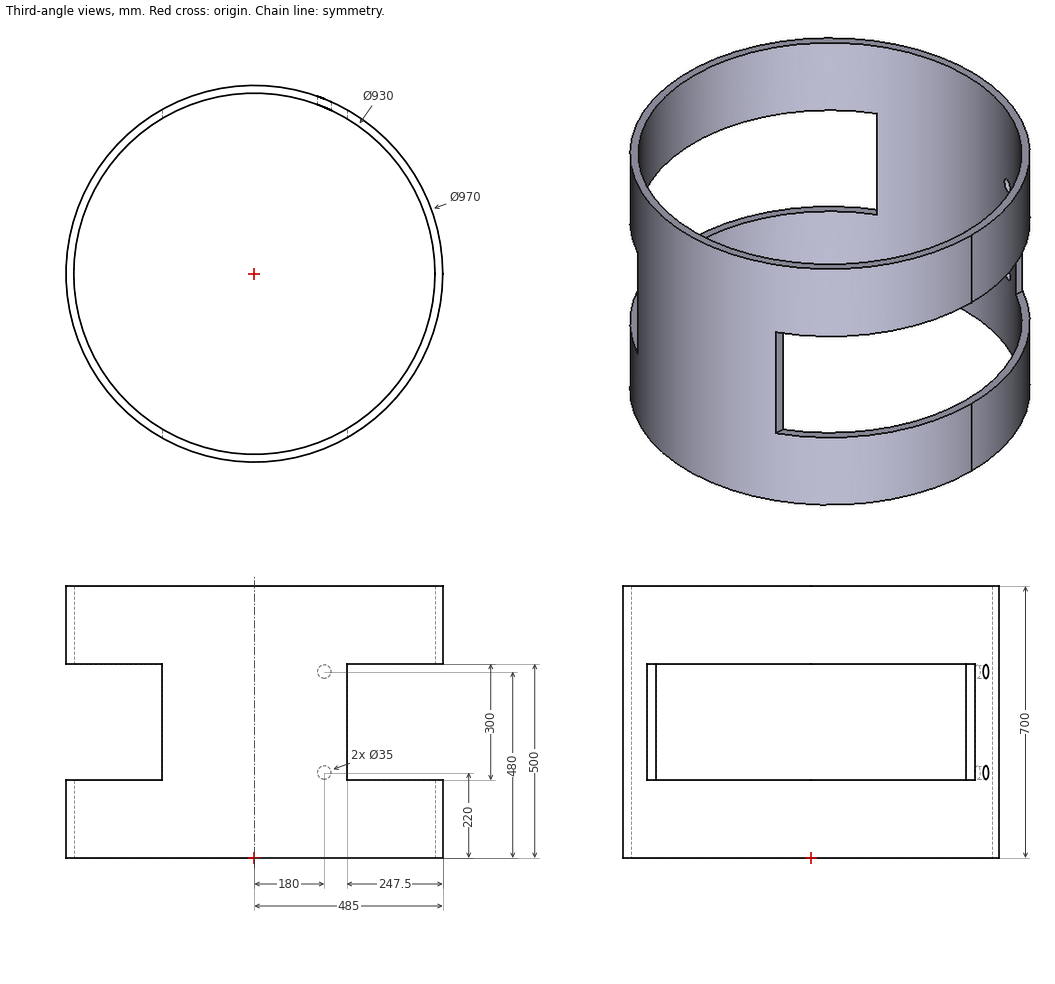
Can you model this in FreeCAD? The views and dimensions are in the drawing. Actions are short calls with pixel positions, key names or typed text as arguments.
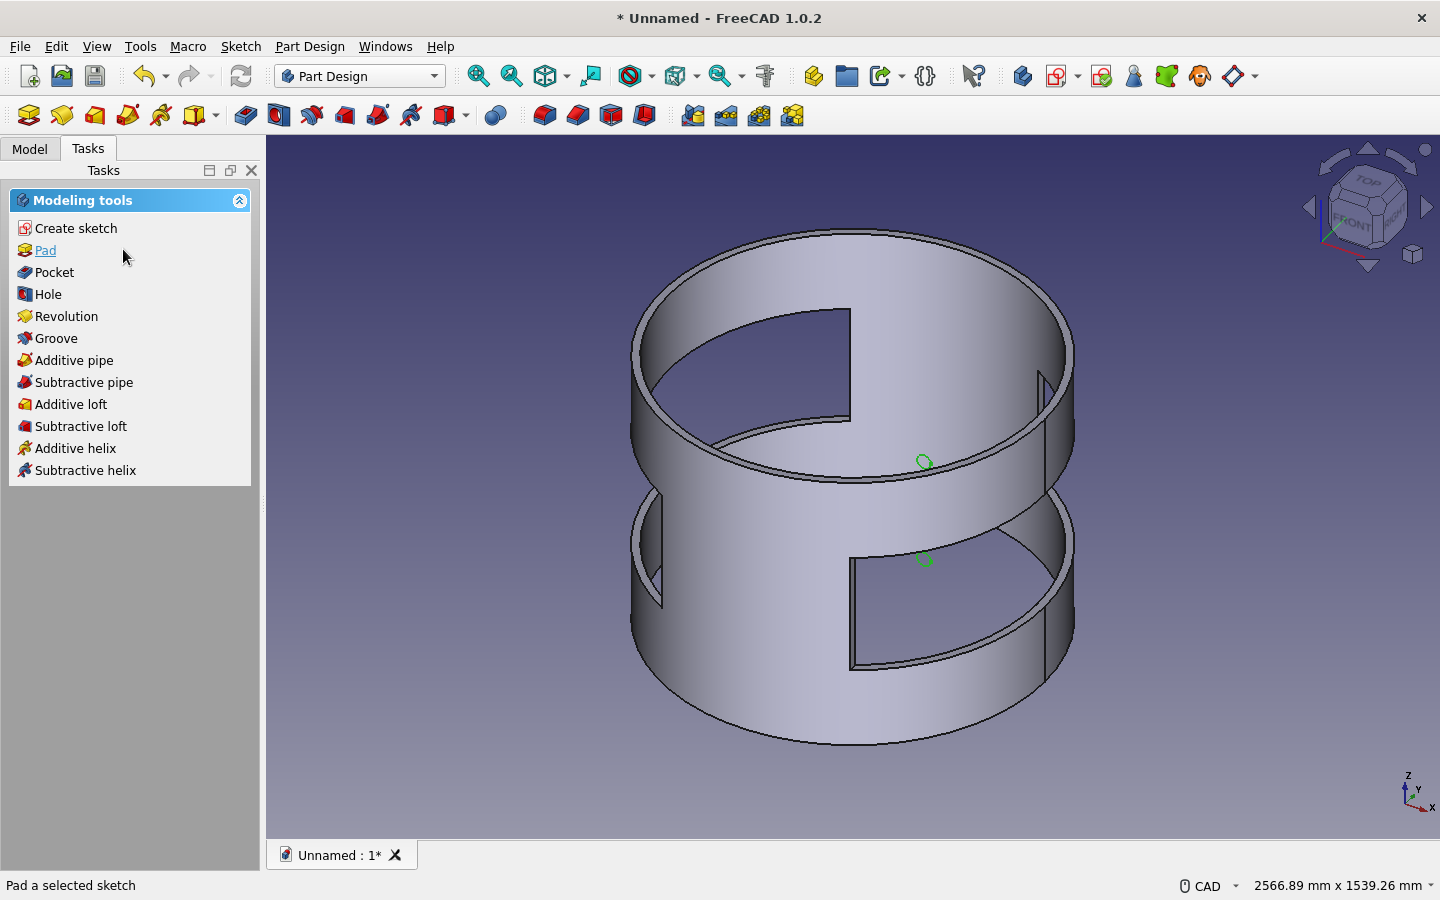
click(246, 116)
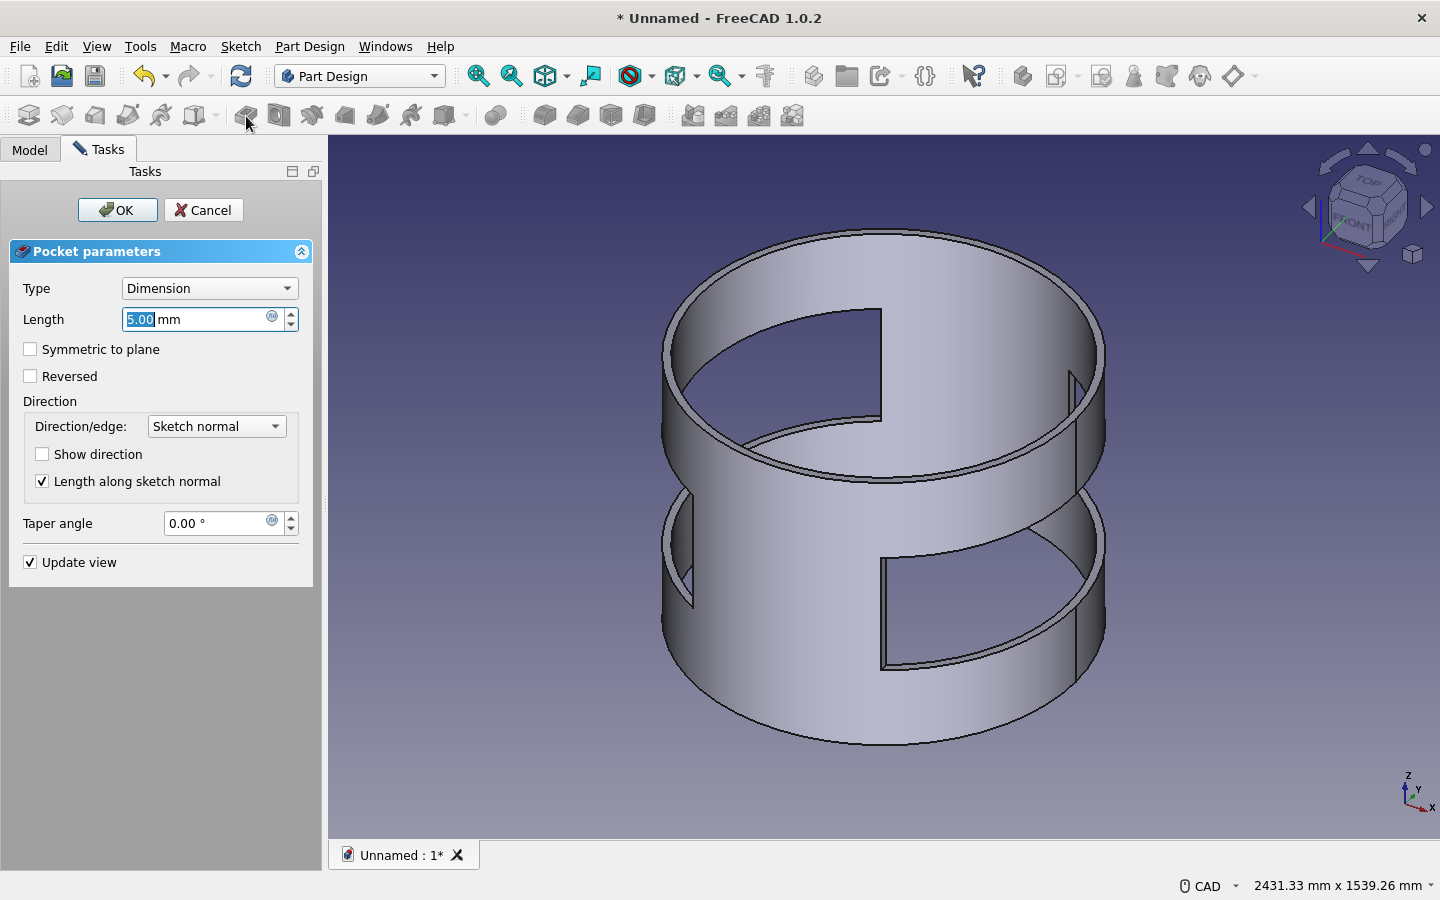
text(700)
key(Tab)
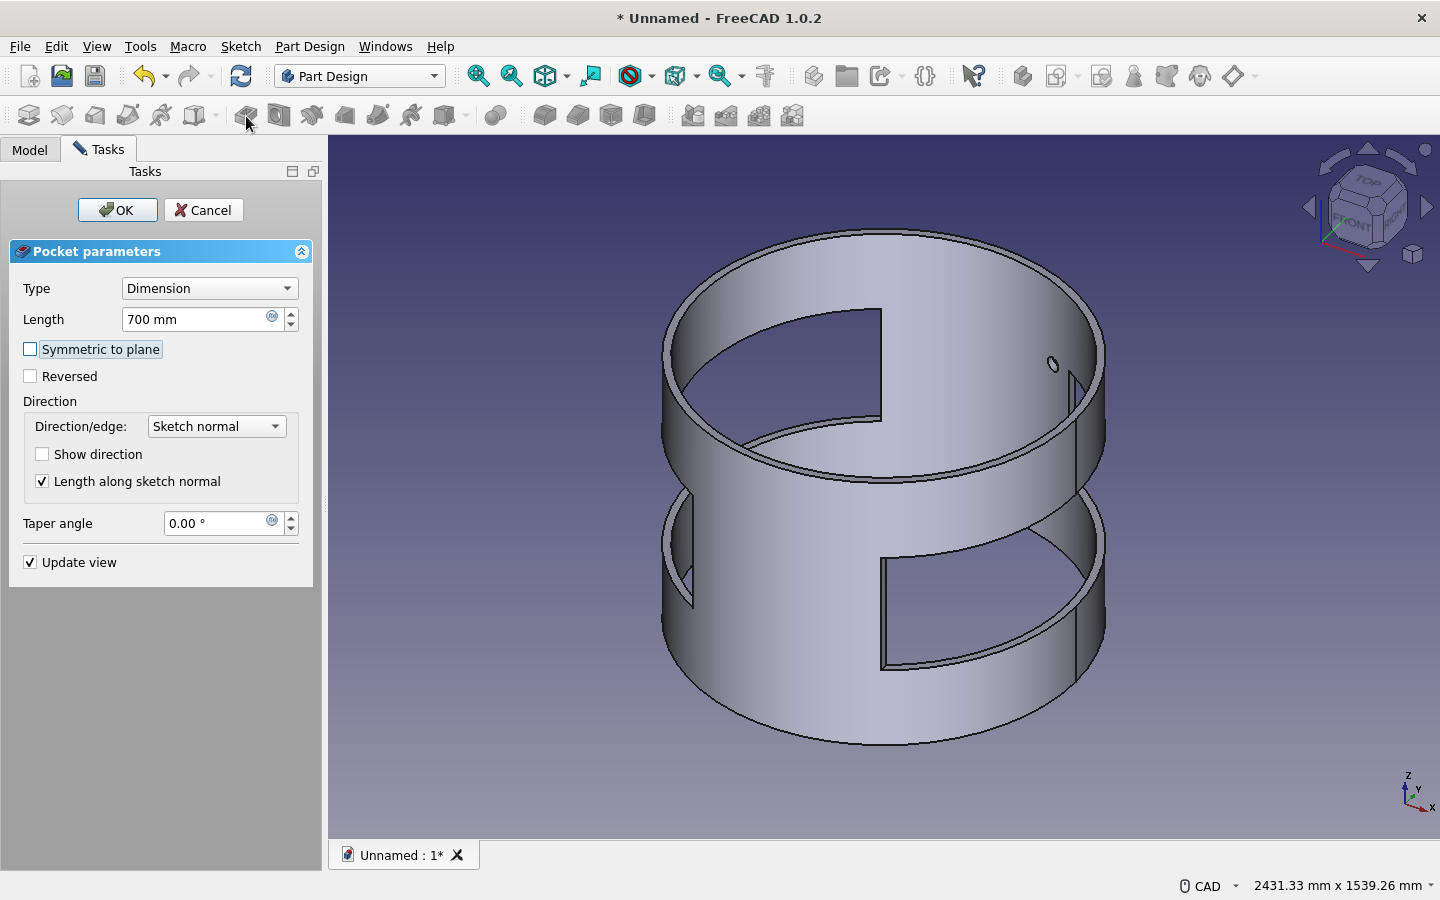
click(118, 210)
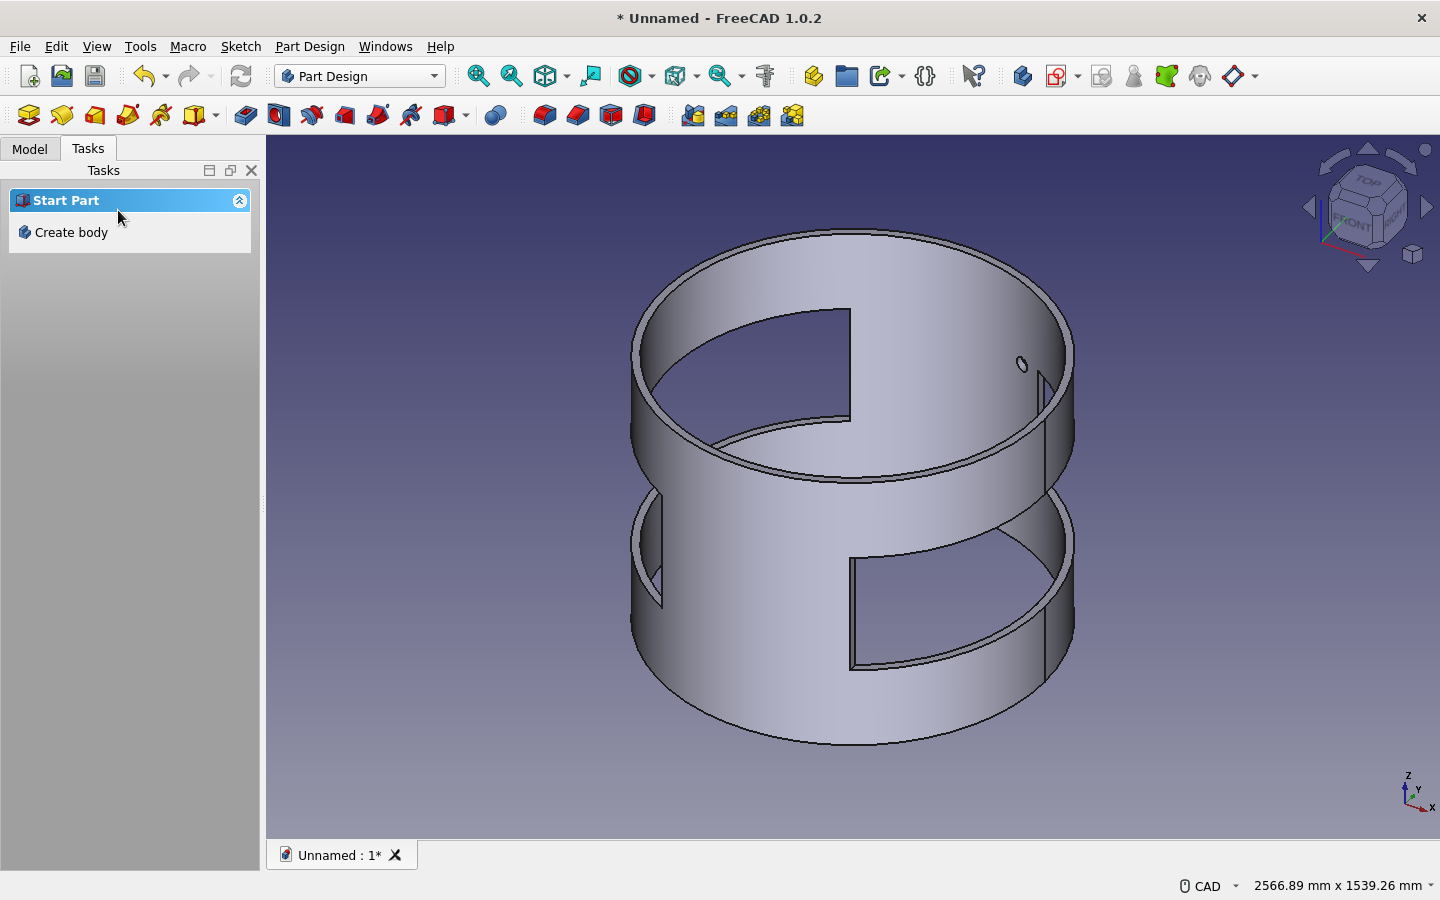
key(0)